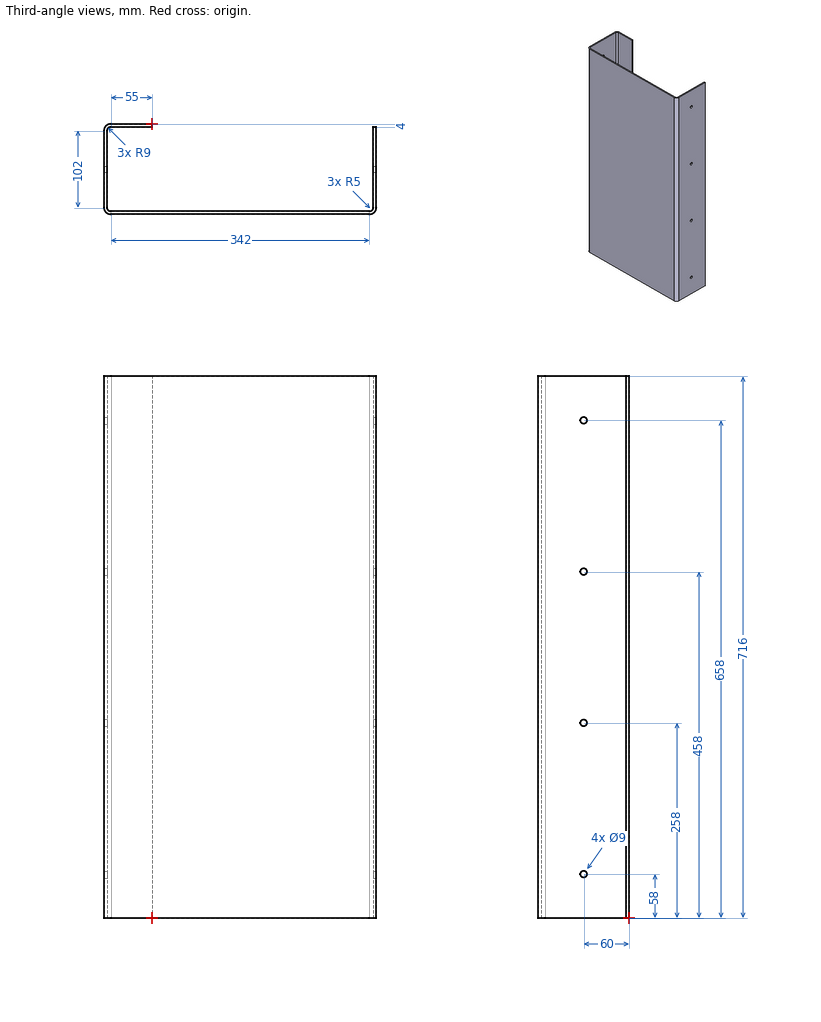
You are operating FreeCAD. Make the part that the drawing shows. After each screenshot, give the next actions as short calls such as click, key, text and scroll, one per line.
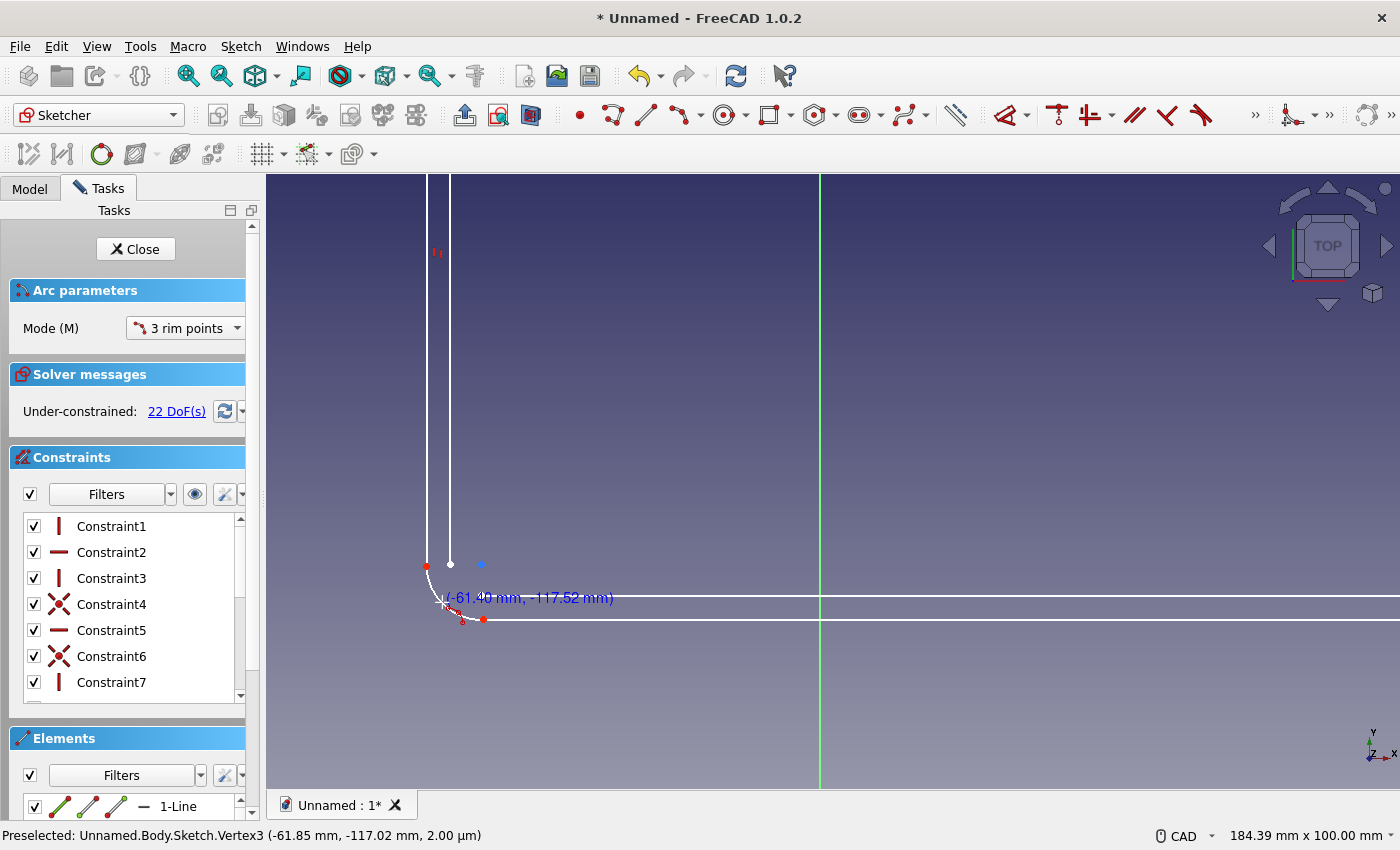
scroll(433, 582, down, 6)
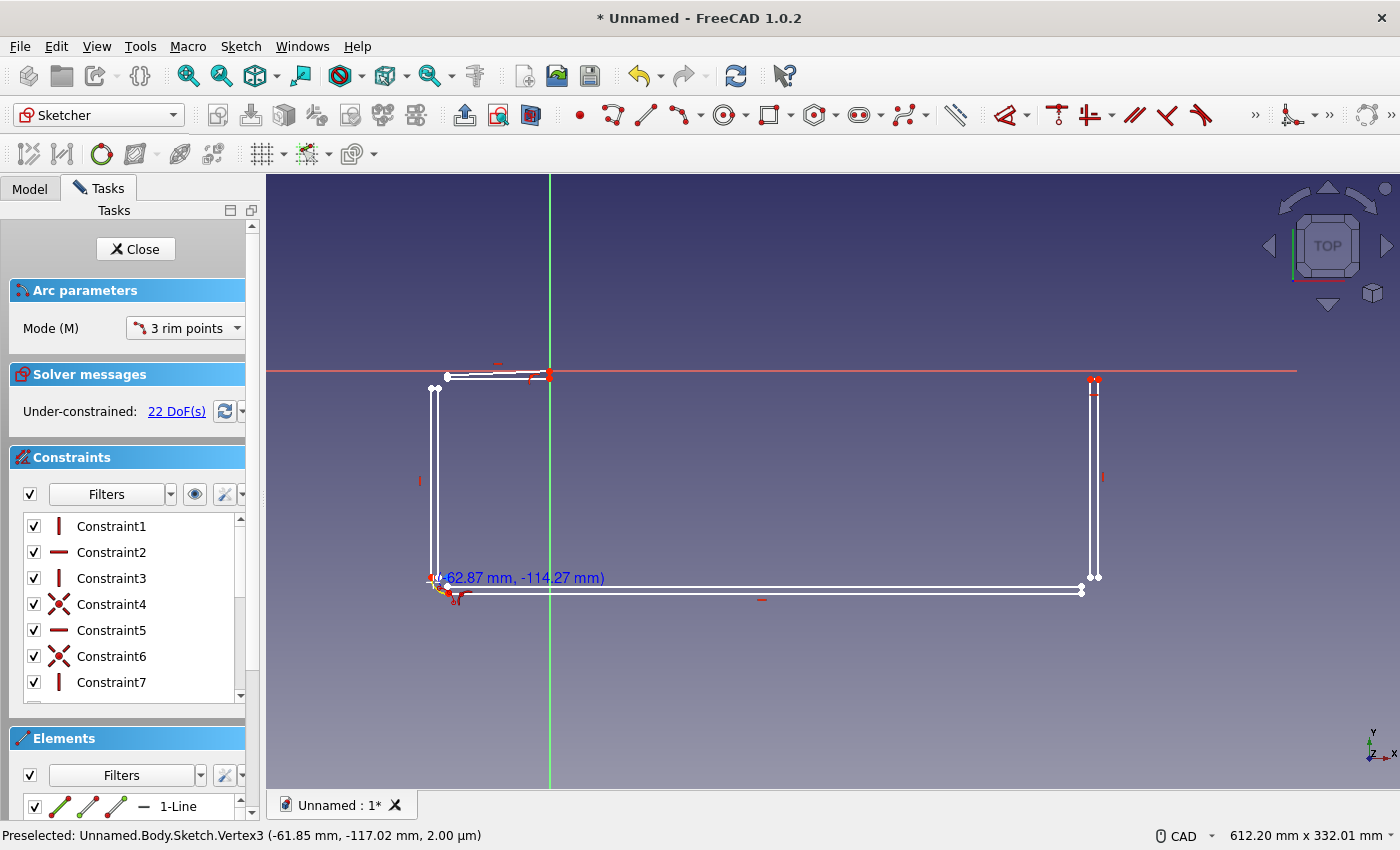
scroll(1081, 593, up, 4)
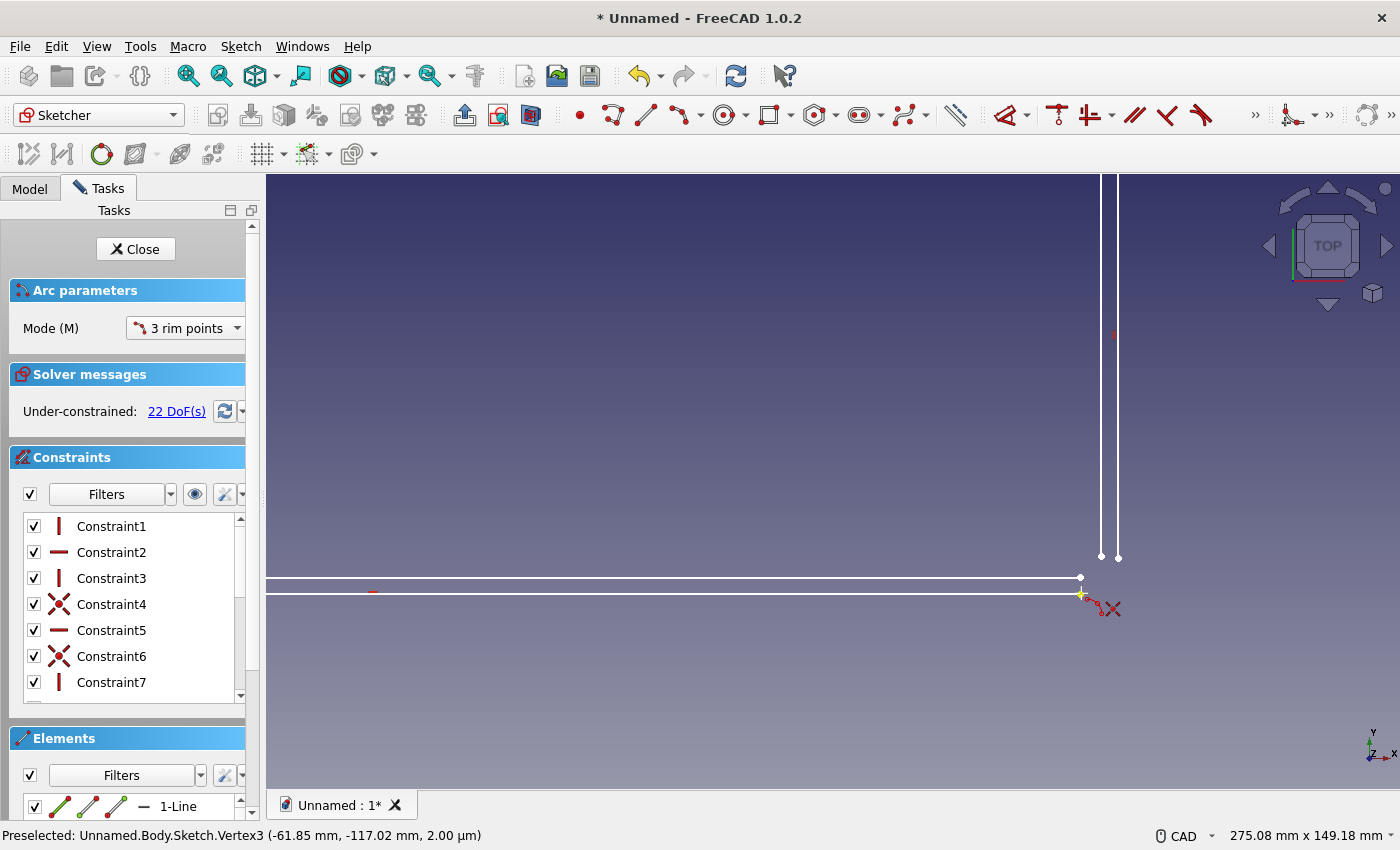
click(1080, 594)
click(1118, 559)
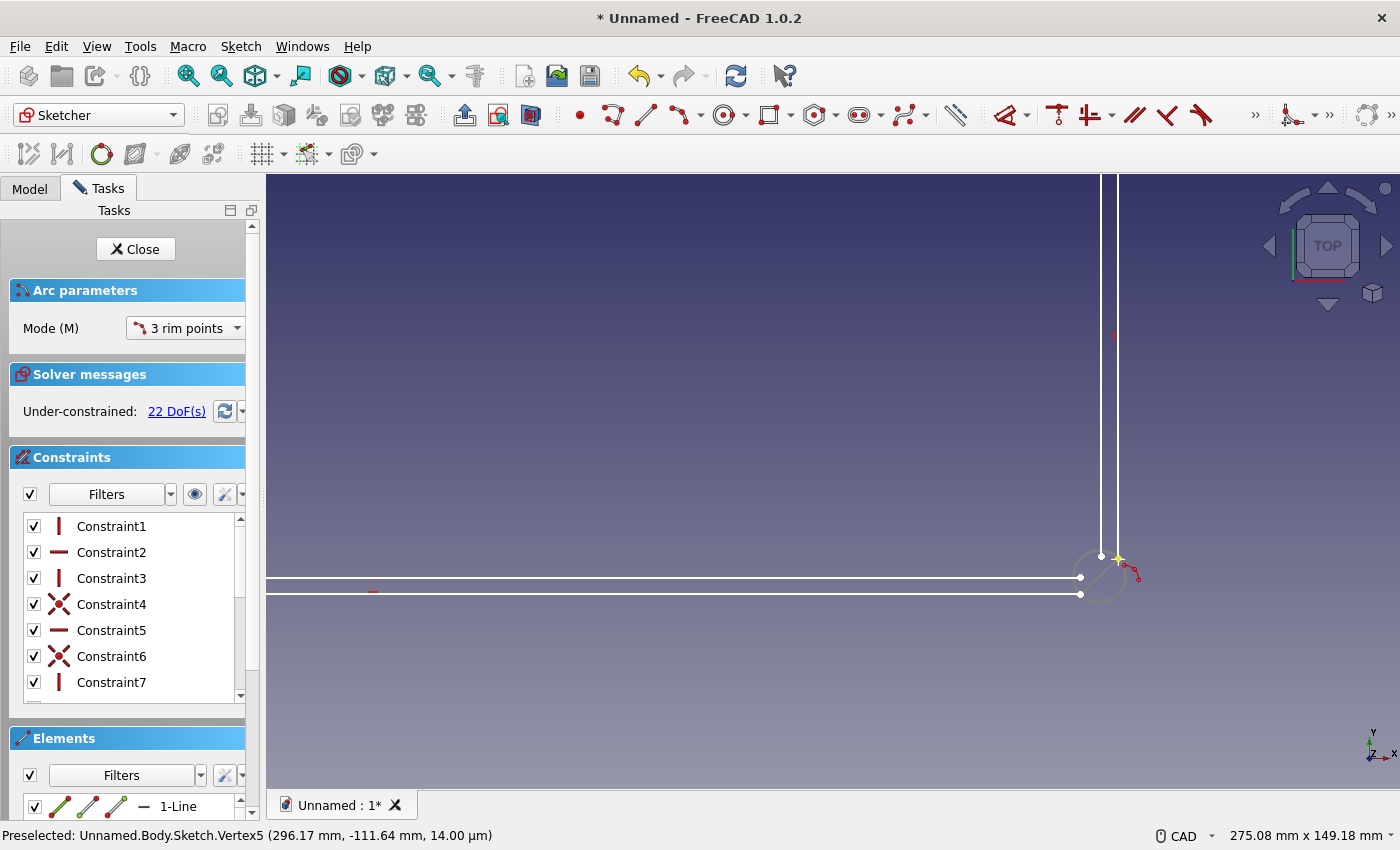
scroll(1107, 582, up, 2)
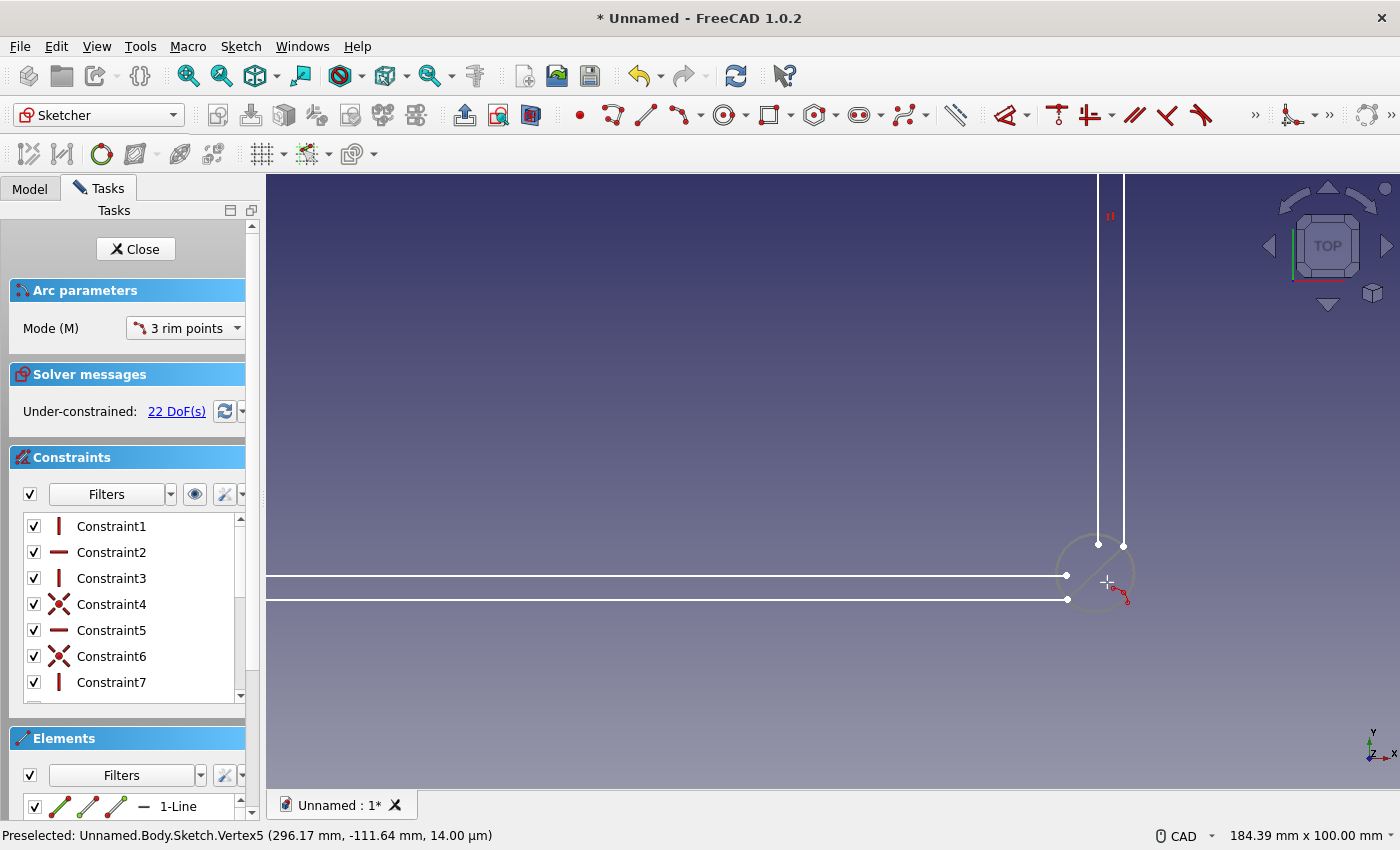
click(1106, 582)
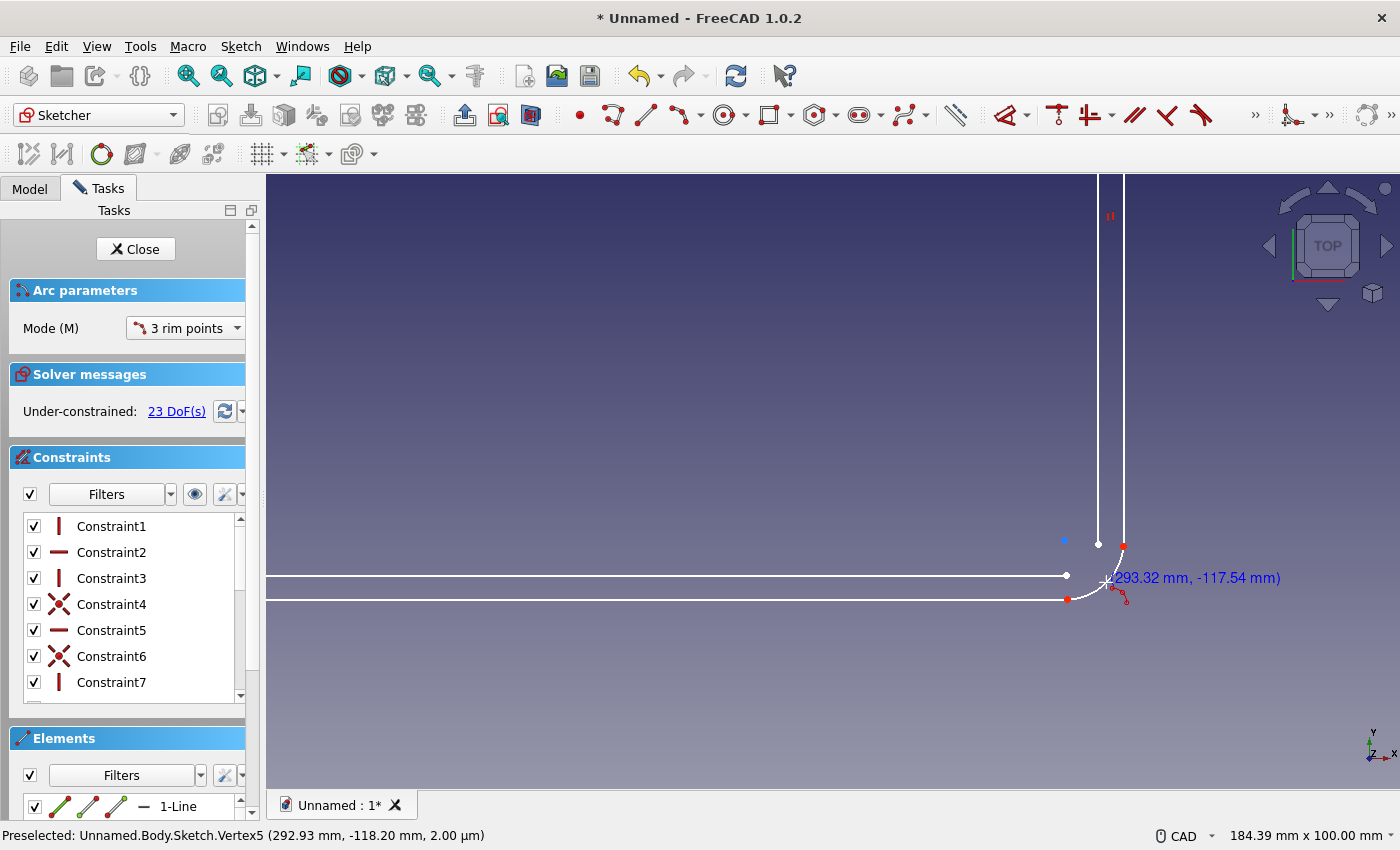
click(1098, 544)
click(1067, 576)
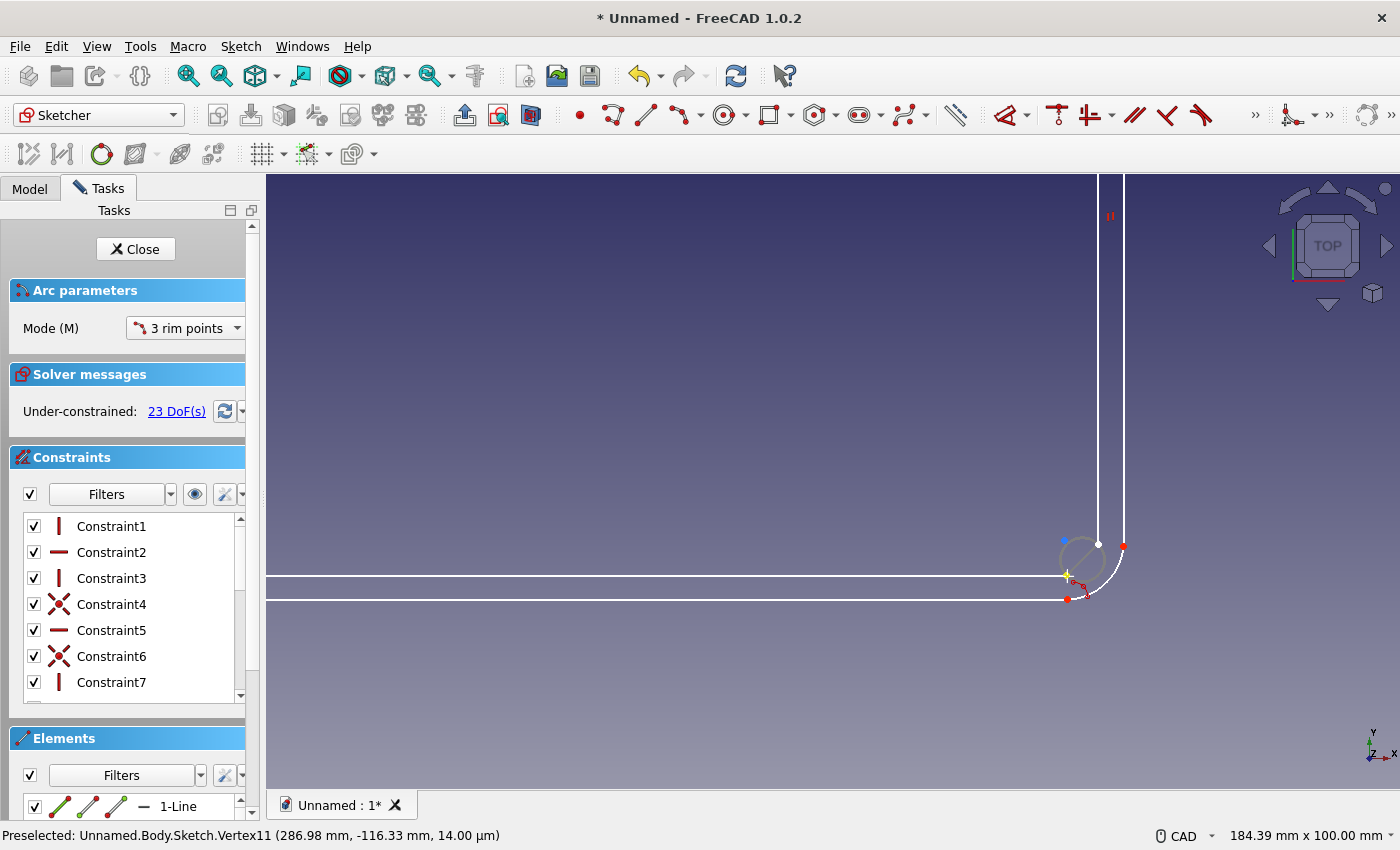
scroll(1089, 565, up, 3)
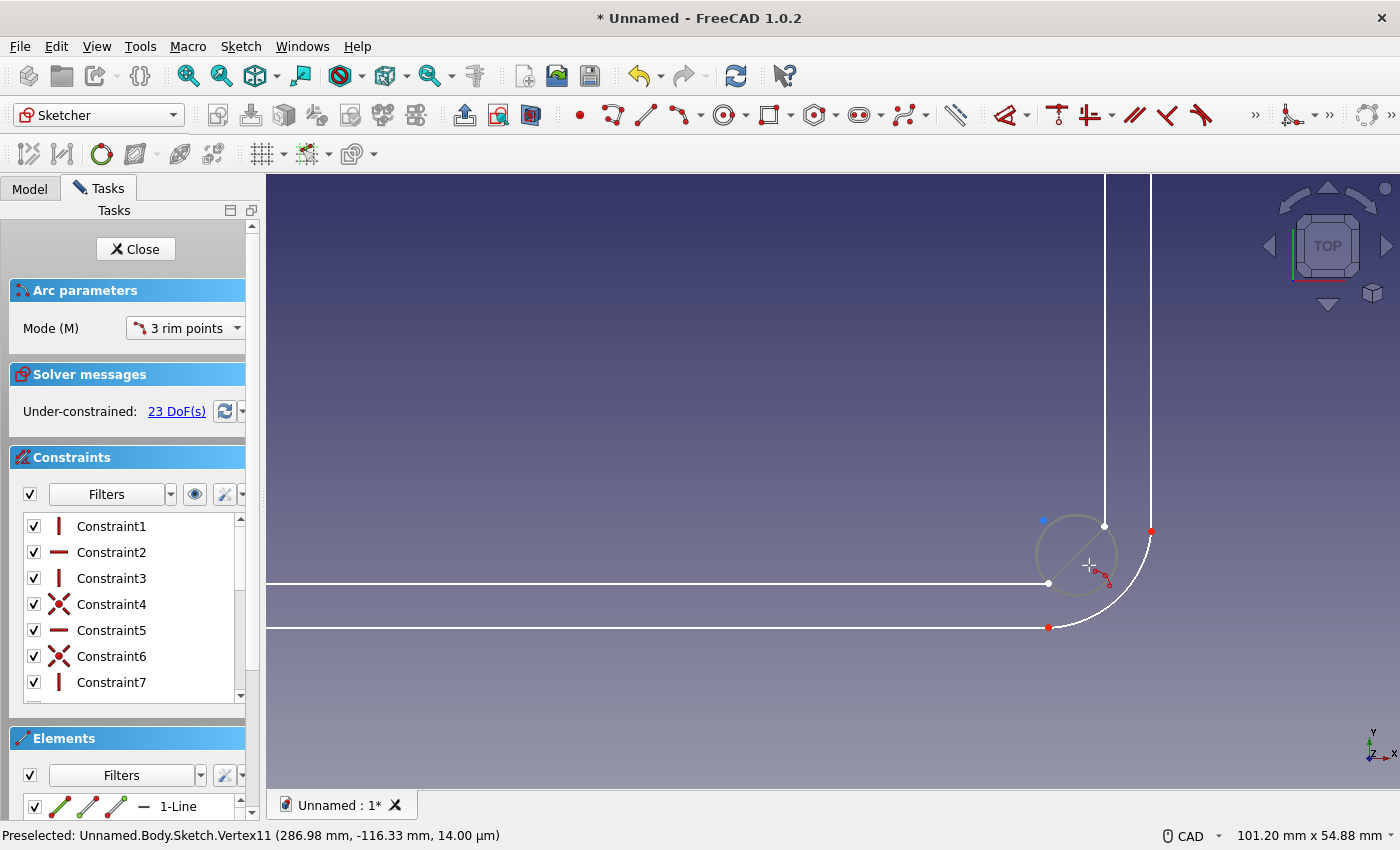
click(1088, 564)